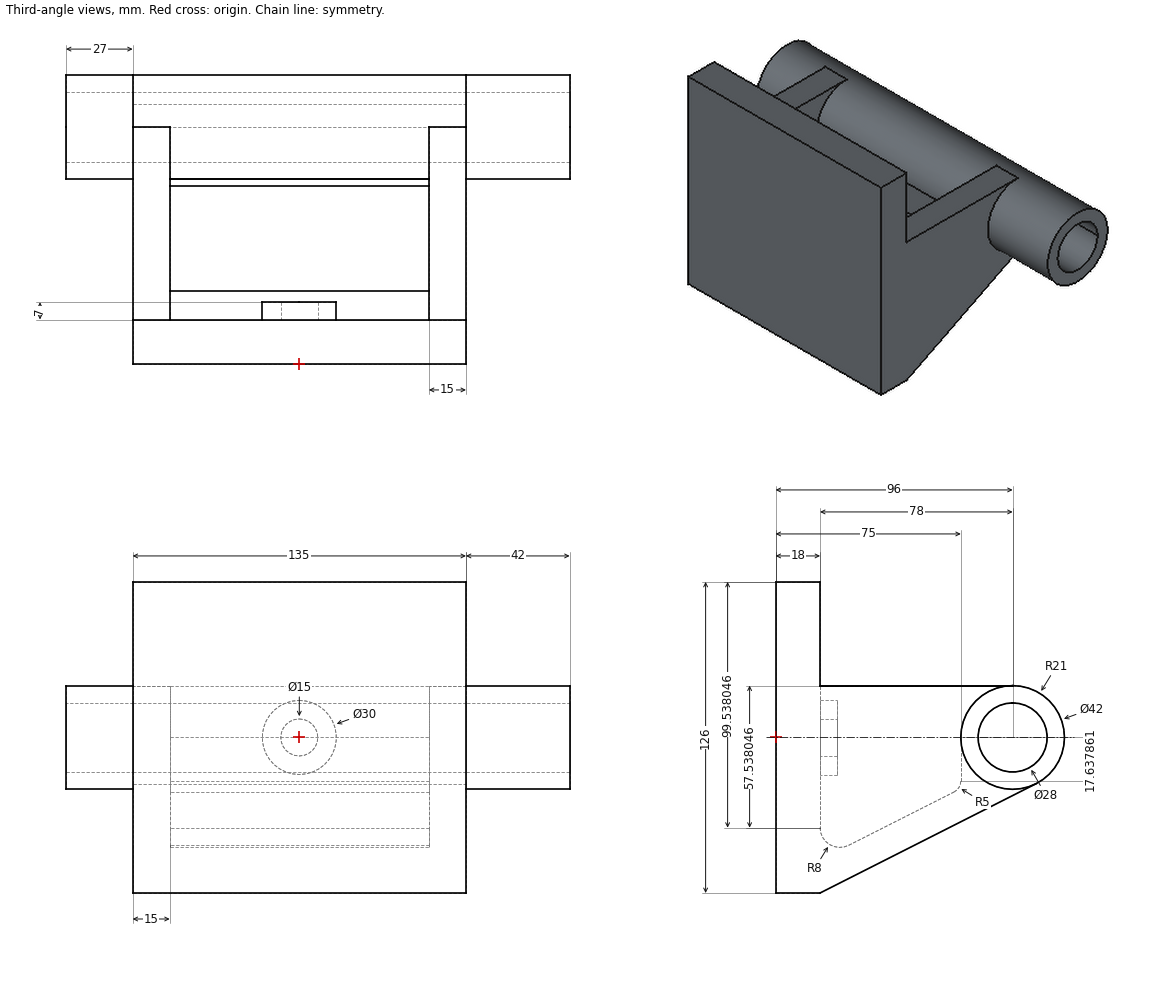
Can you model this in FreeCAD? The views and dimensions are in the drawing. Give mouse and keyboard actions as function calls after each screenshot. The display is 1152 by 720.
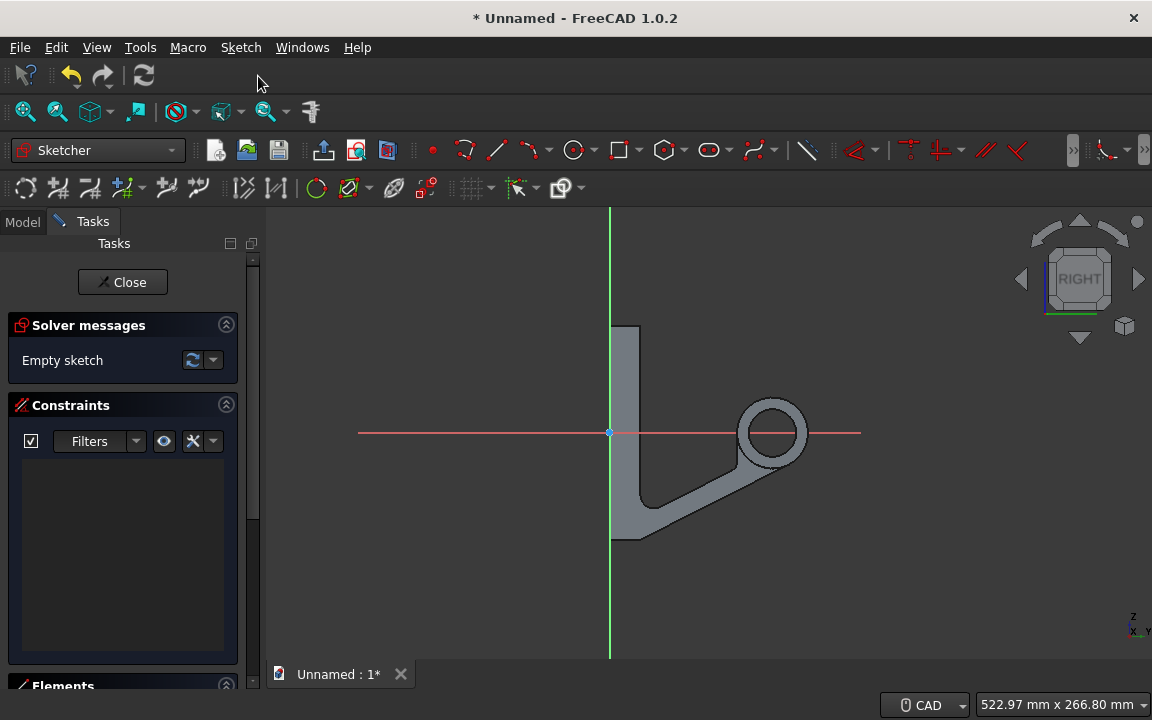
click(388, 150)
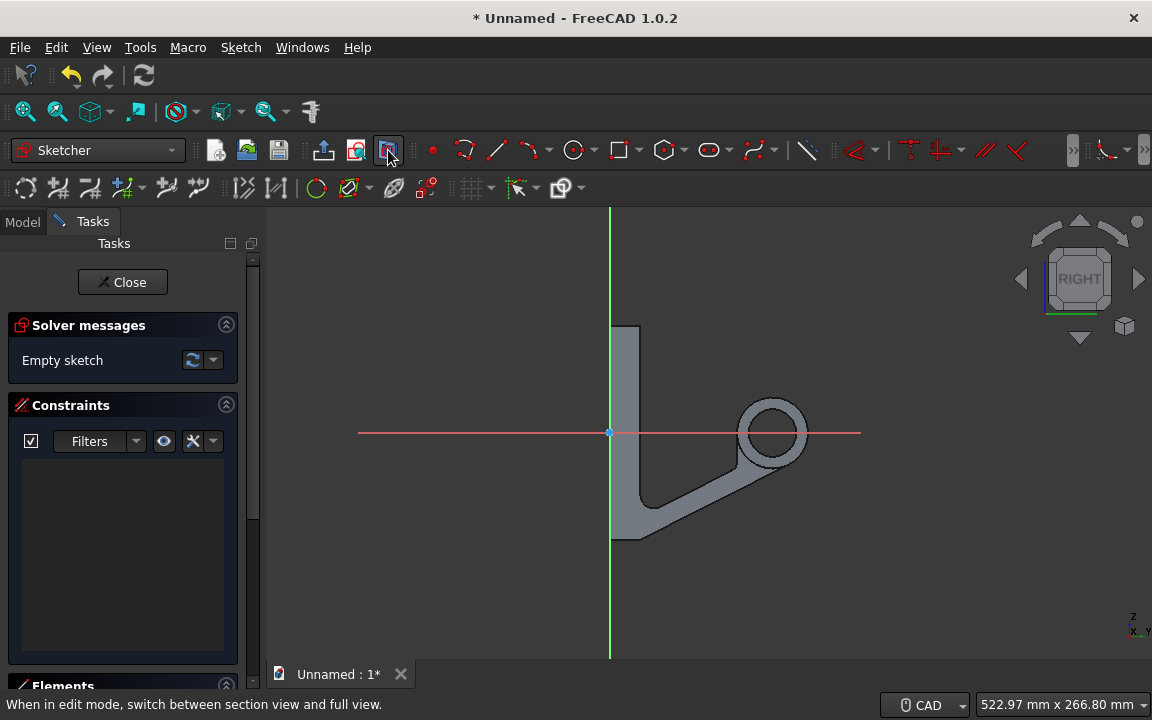
scroll(721, 463, up, 5)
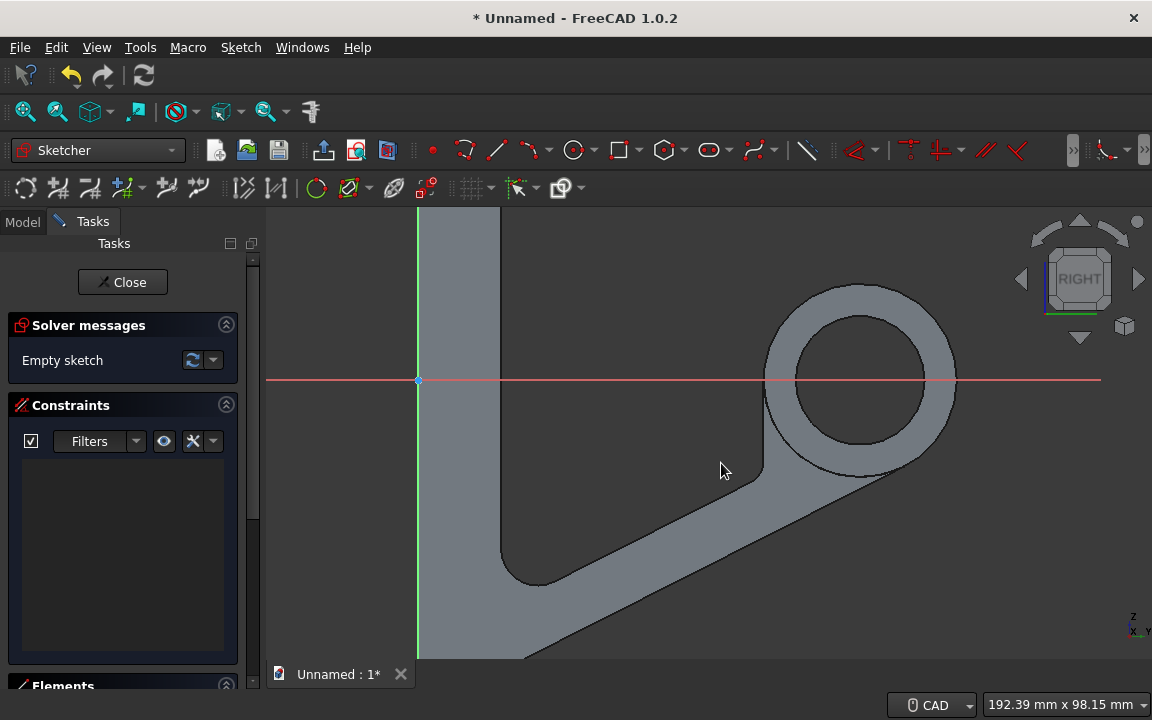
click(466, 150)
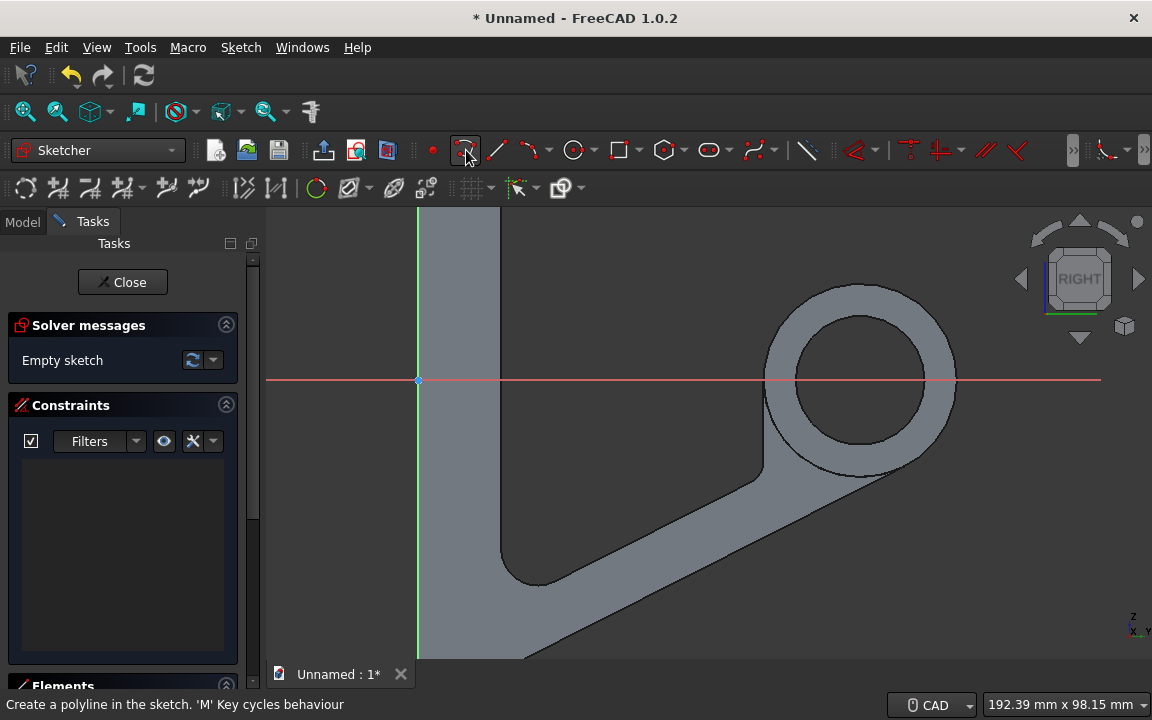
click(860, 284)
click(501, 284)
click(501, 549)
right_click(501, 549)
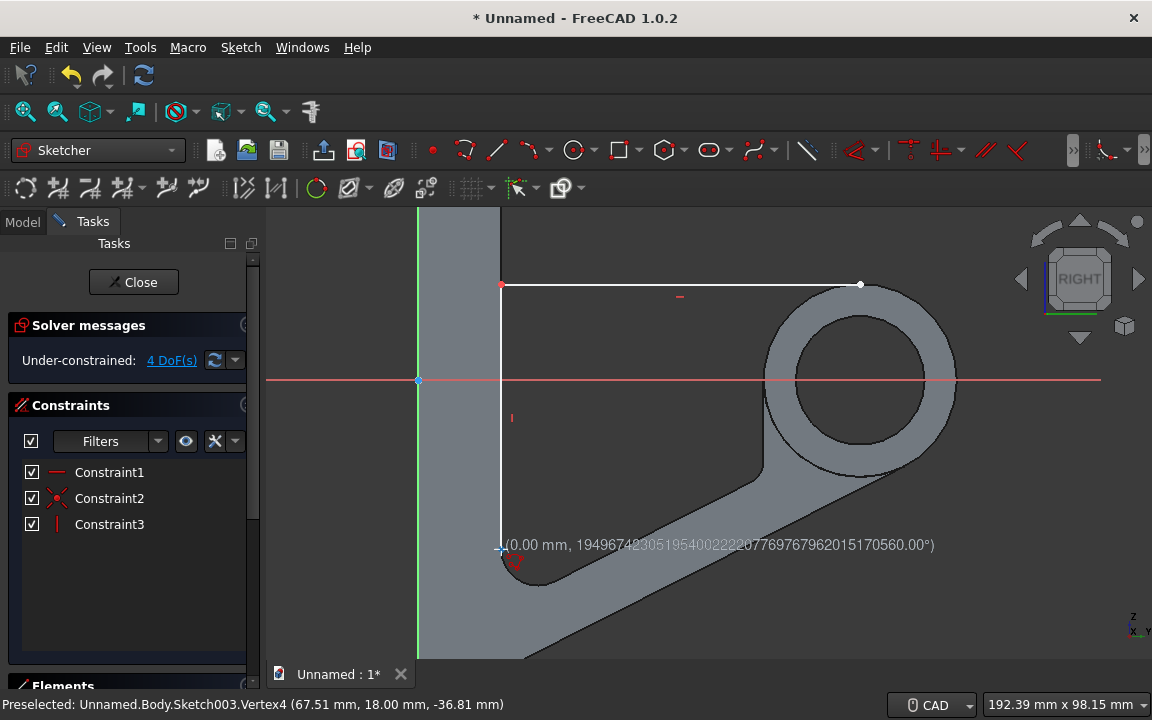
click(498, 150)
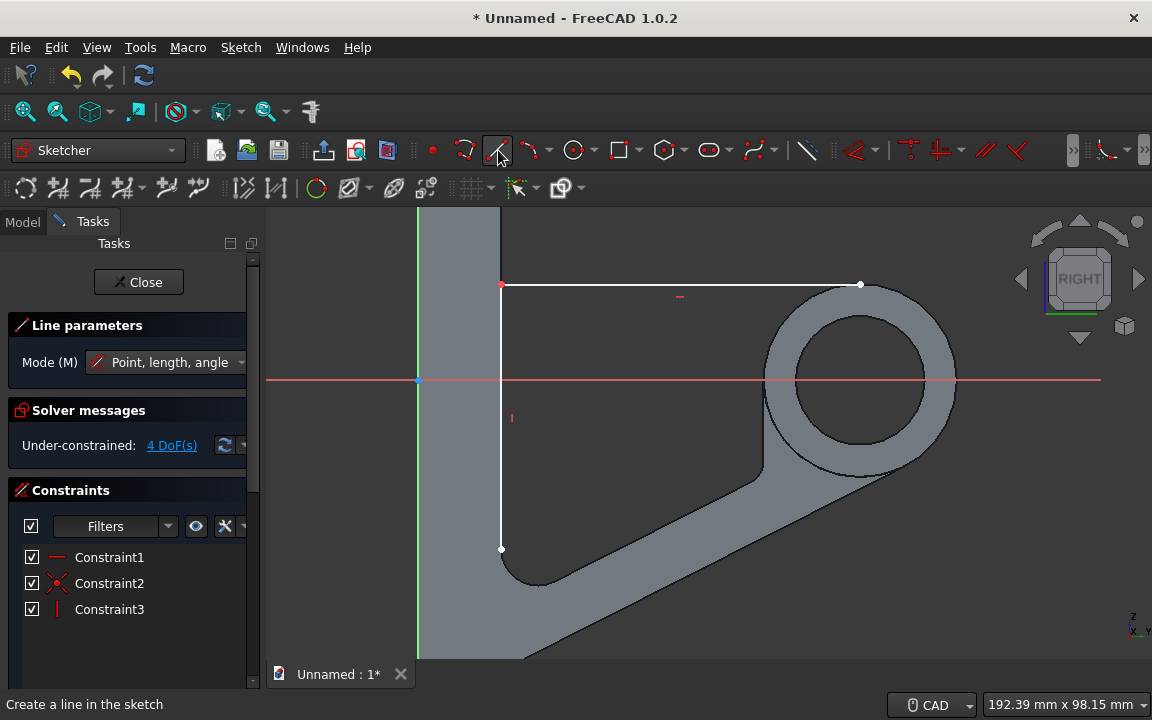
click(554, 582)
click(751, 482)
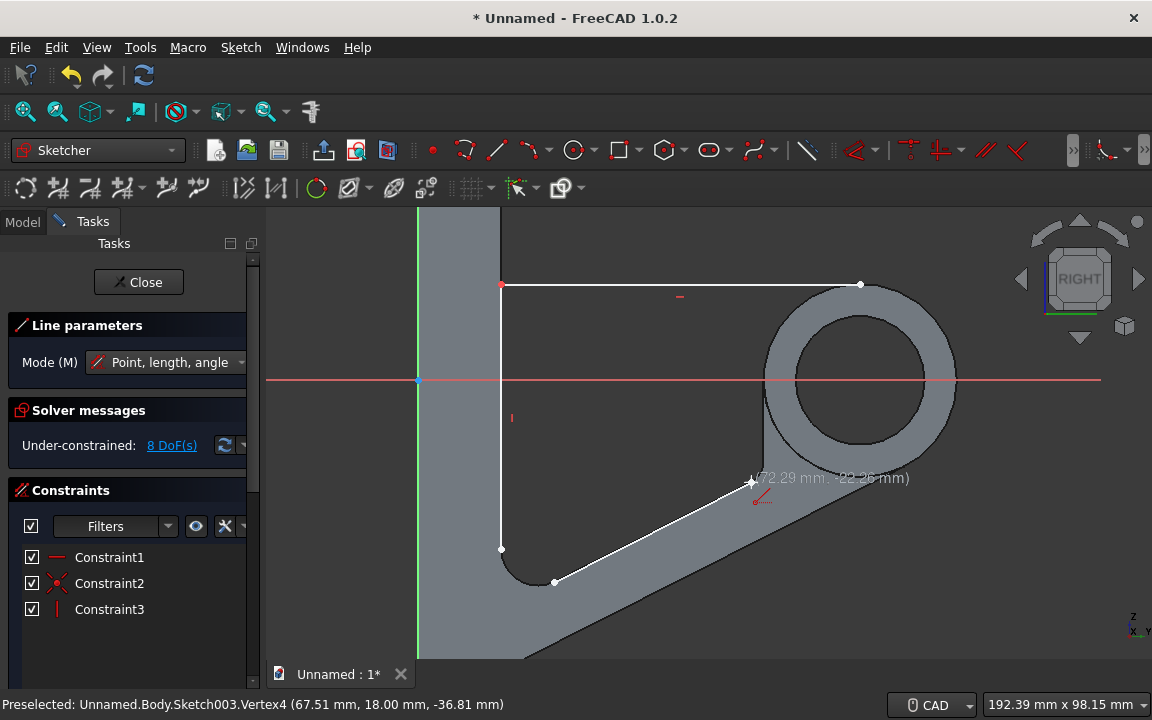
click(763, 462)
click(763, 380)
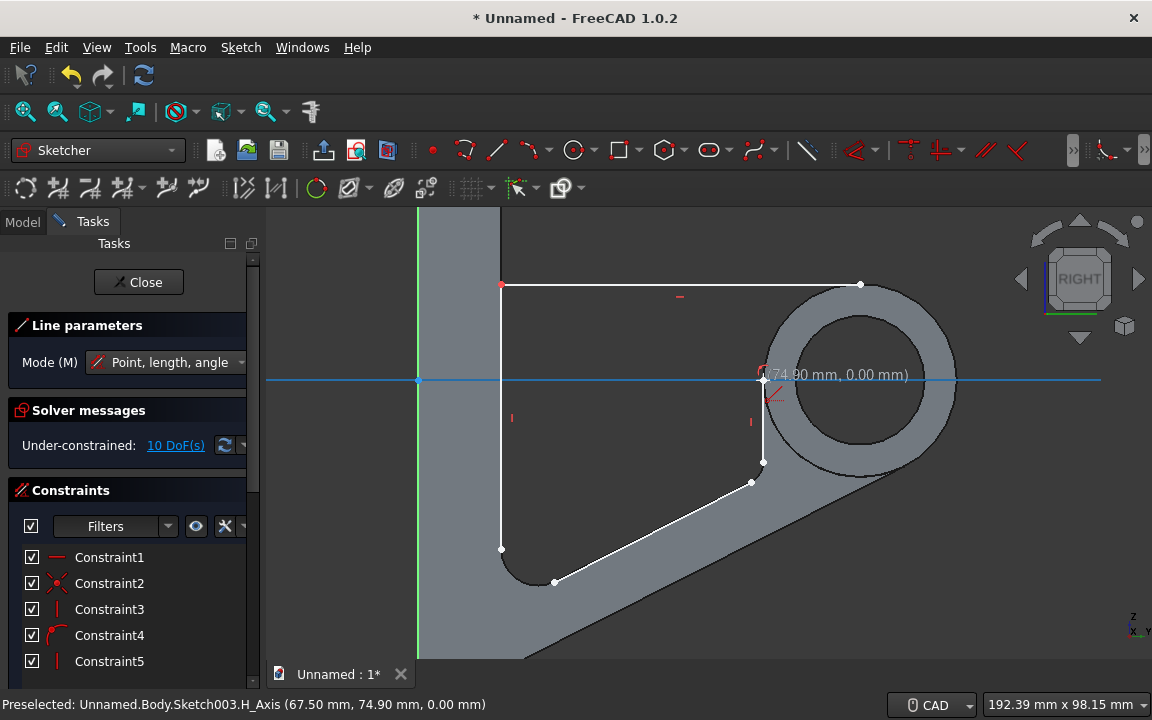
click(530, 150)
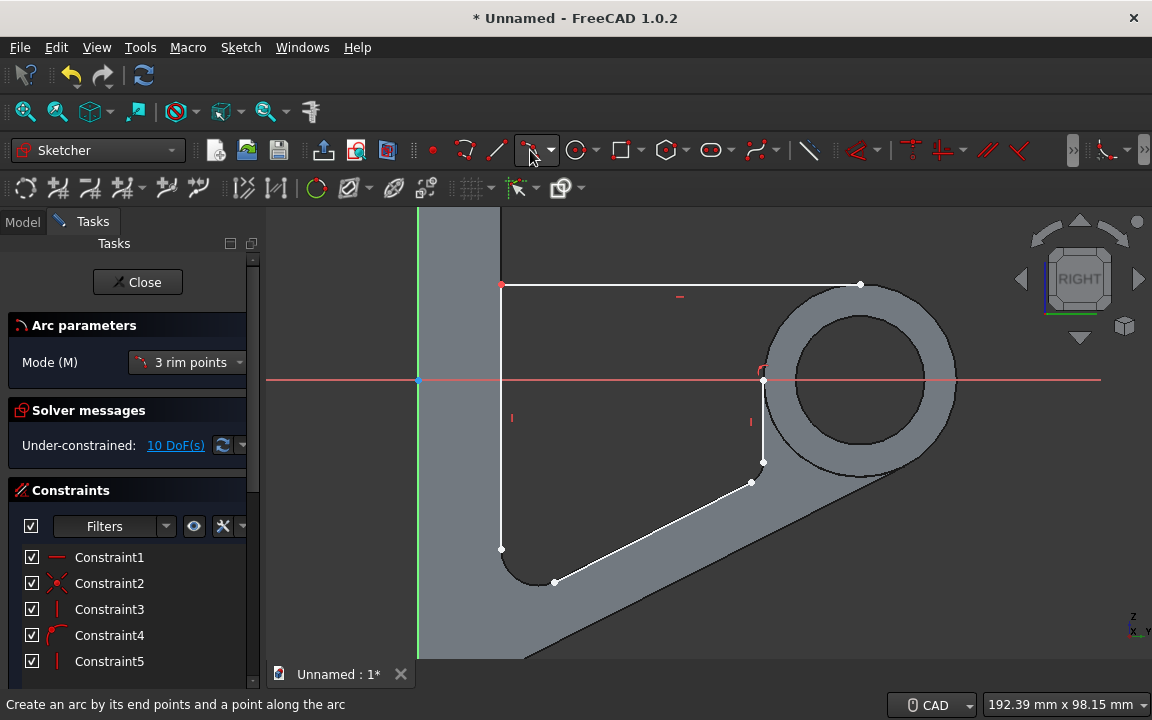
click(501, 550)
click(554, 583)
click(519, 580)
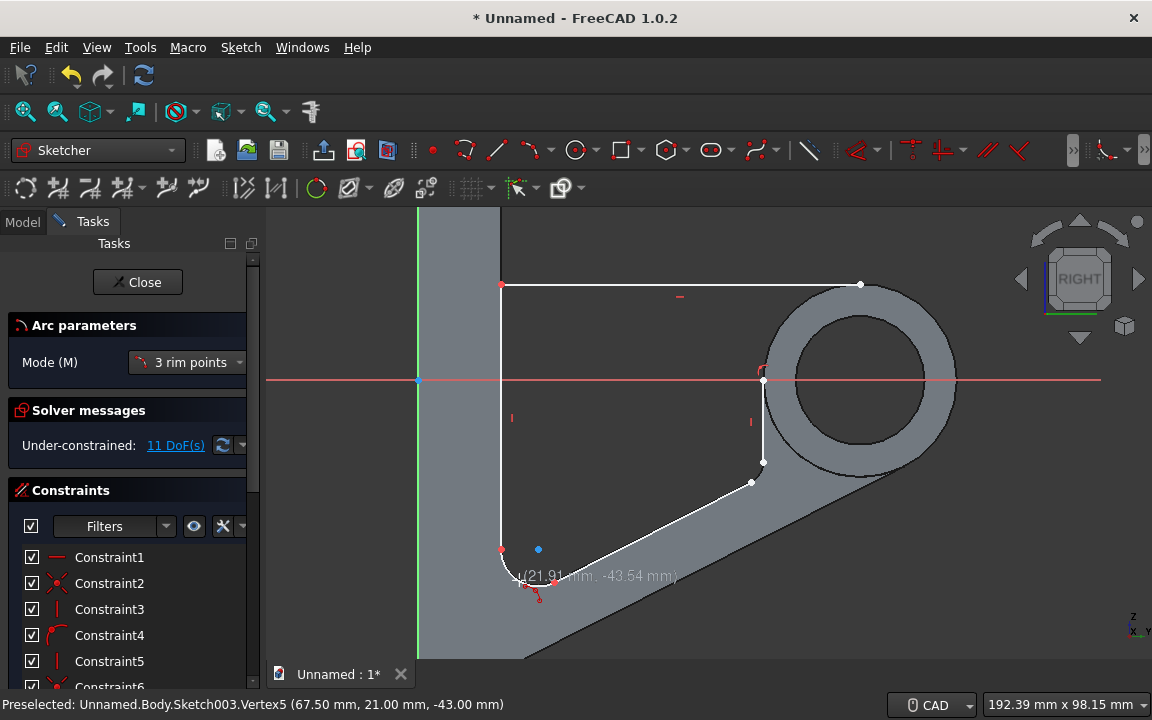
click(751, 483)
click(763, 463)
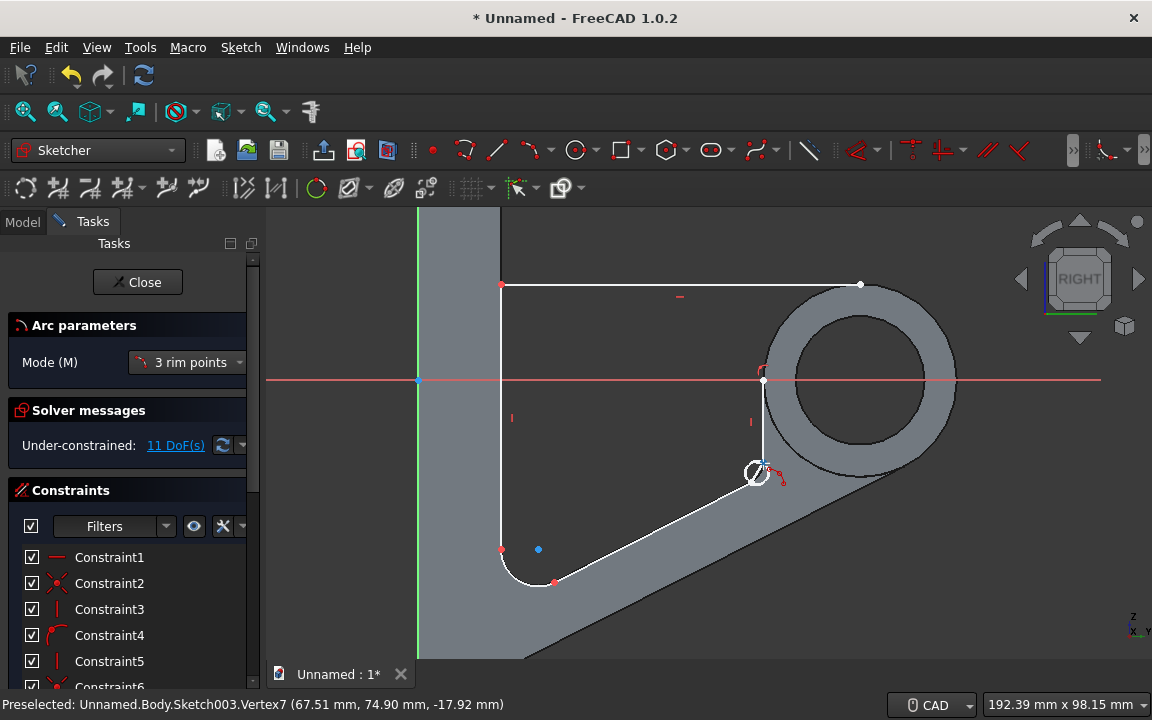
scroll(760, 474, up, 8)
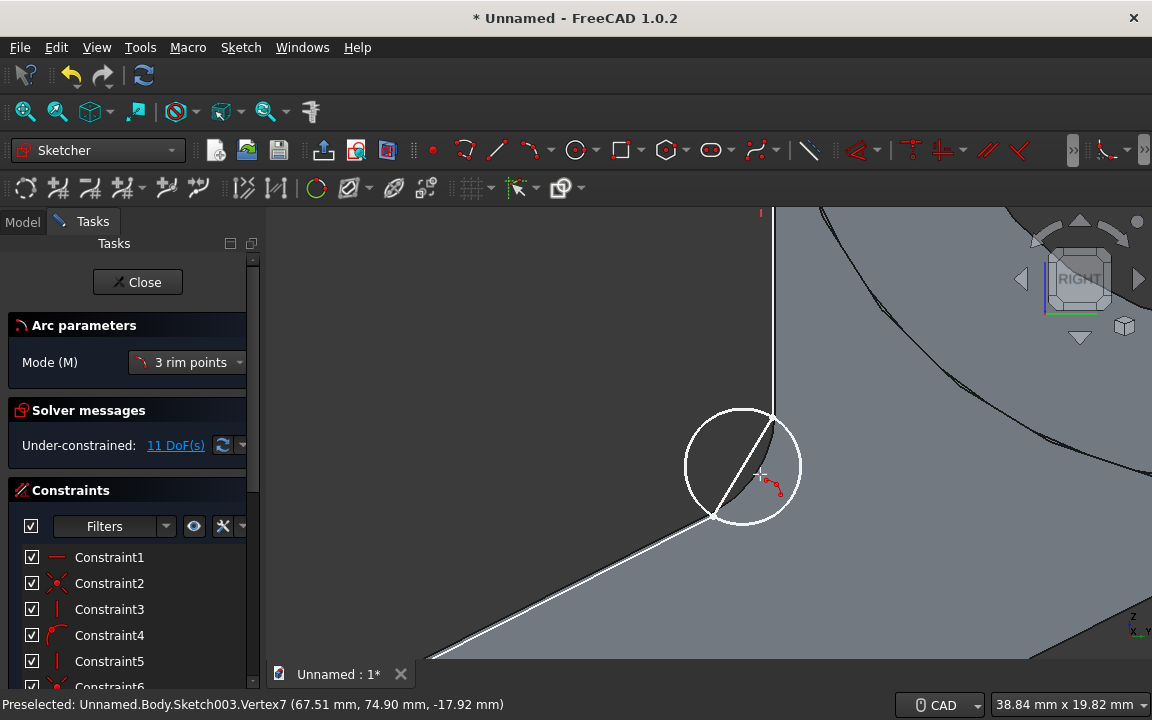
click(758, 470)